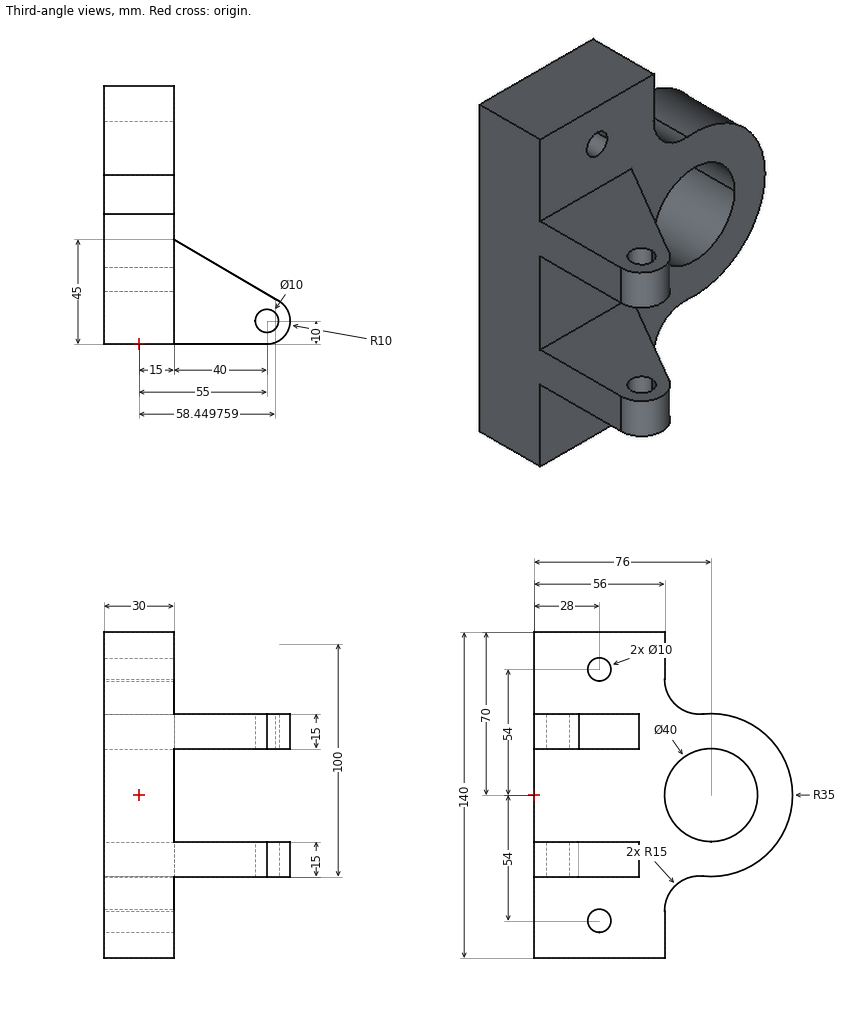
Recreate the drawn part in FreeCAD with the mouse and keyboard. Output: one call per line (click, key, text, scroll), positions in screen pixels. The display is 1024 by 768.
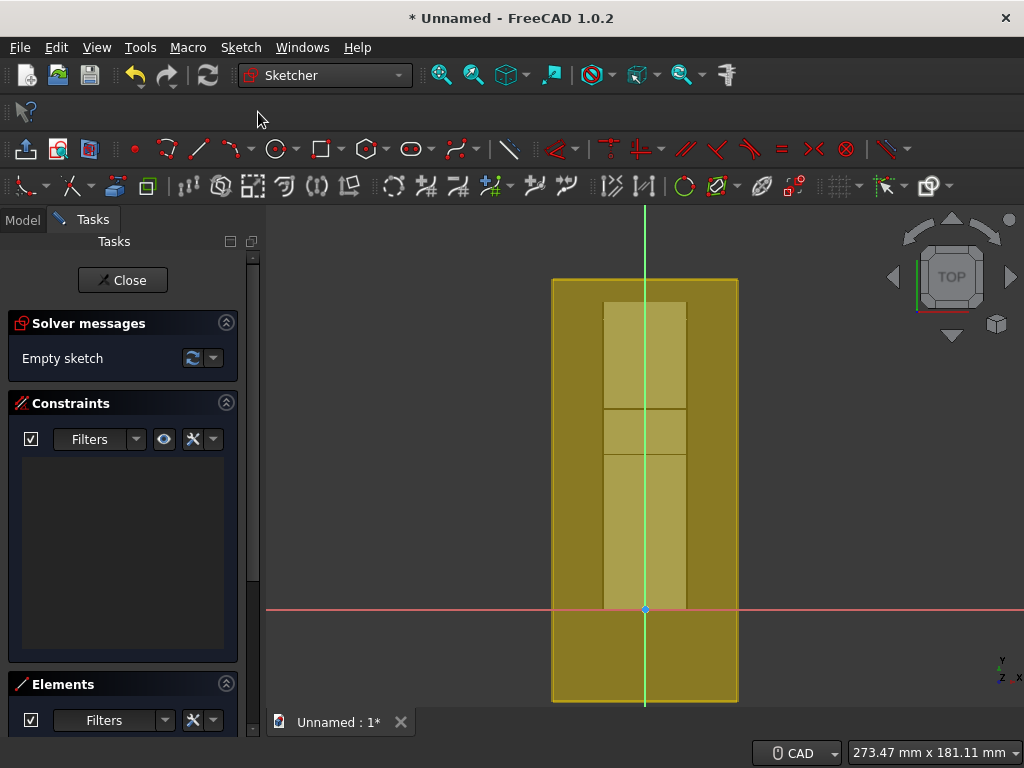
scroll(859, 622, up, 4)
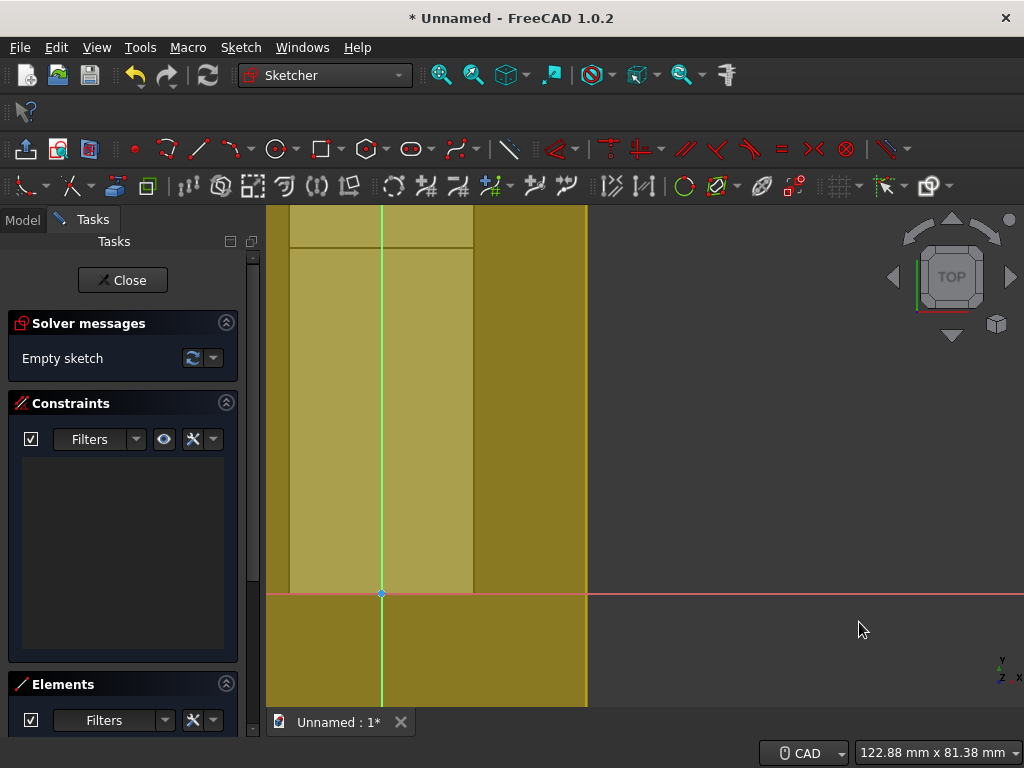
click(168, 150)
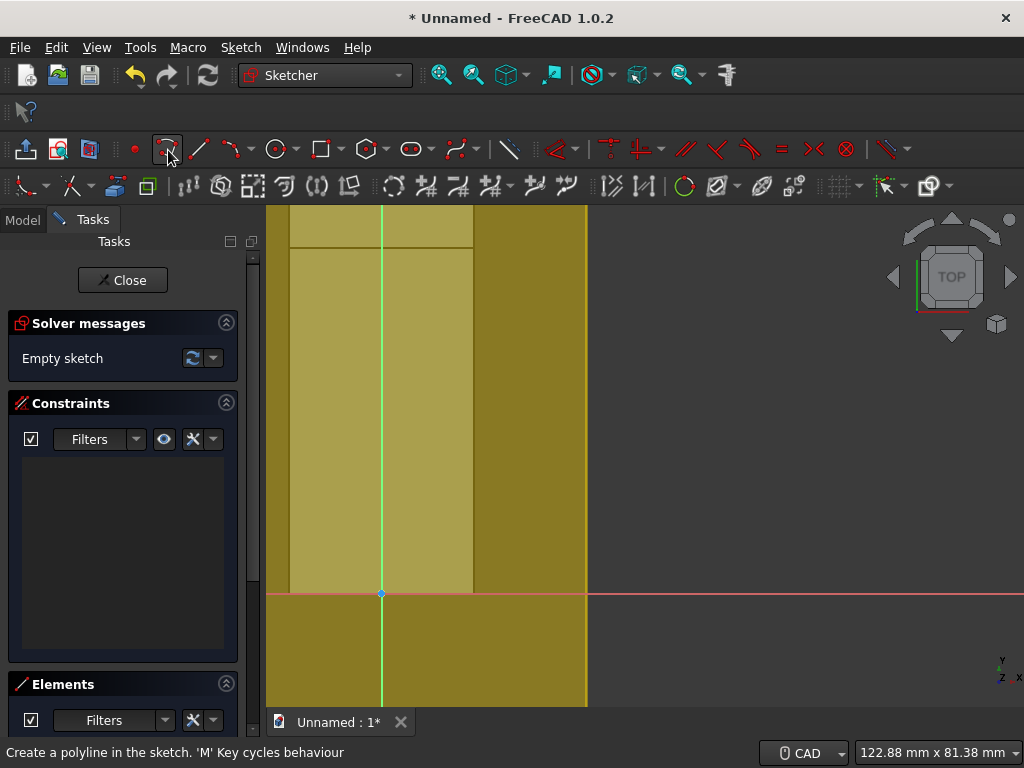
click(742, 474)
click(474, 316)
click(474, 594)
click(721, 585)
right_click(721, 585)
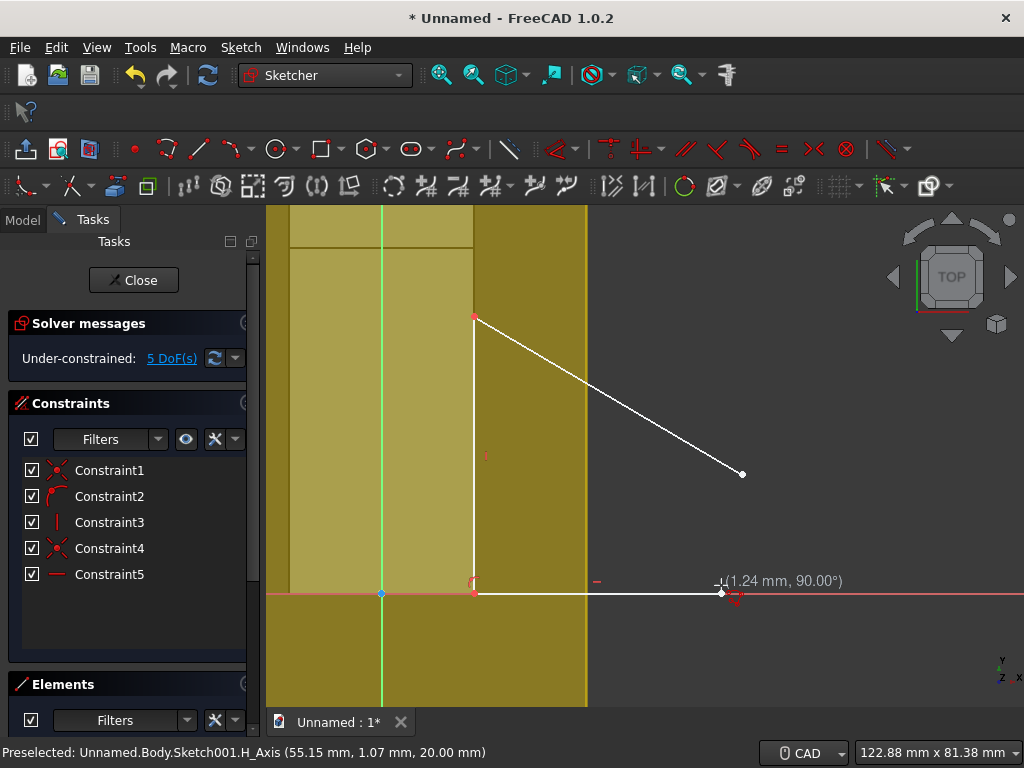
key(g)
key(3)
key(a)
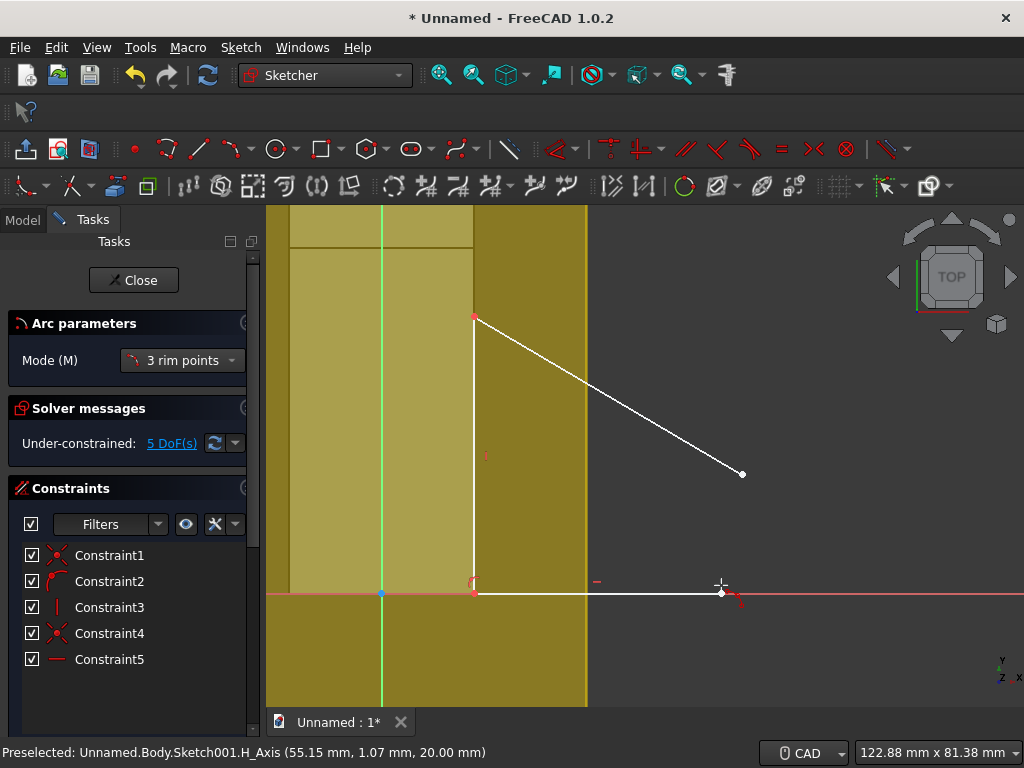
click(721, 594)
click(742, 475)
click(782, 543)
key(Escape)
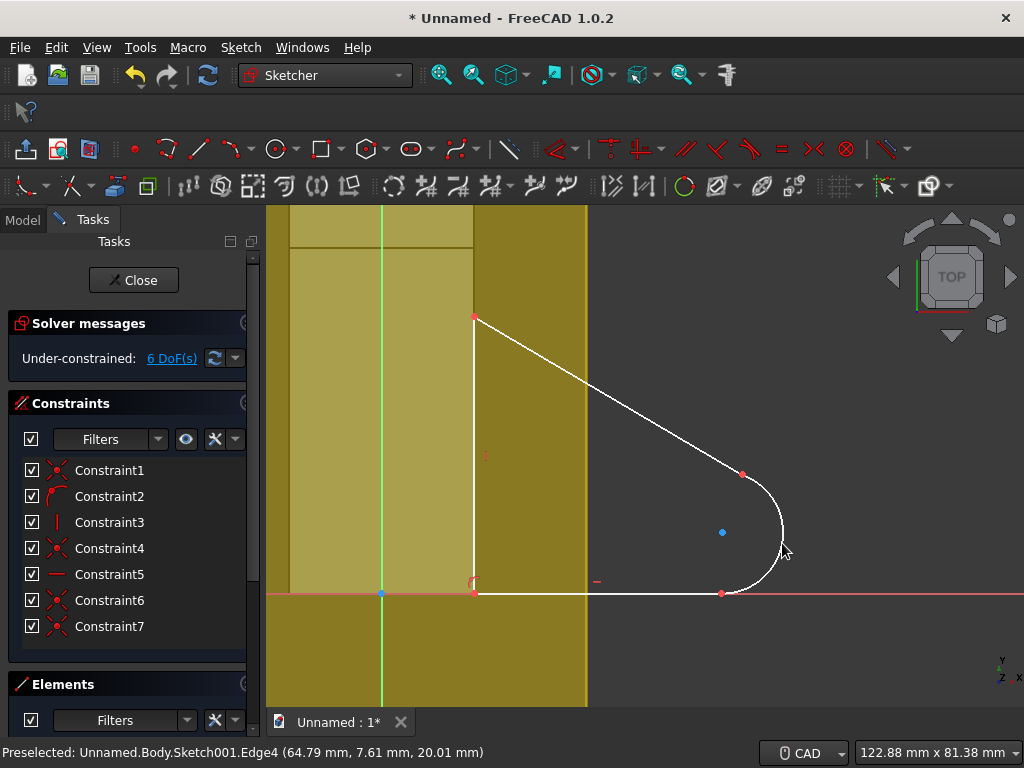
click(548, 594)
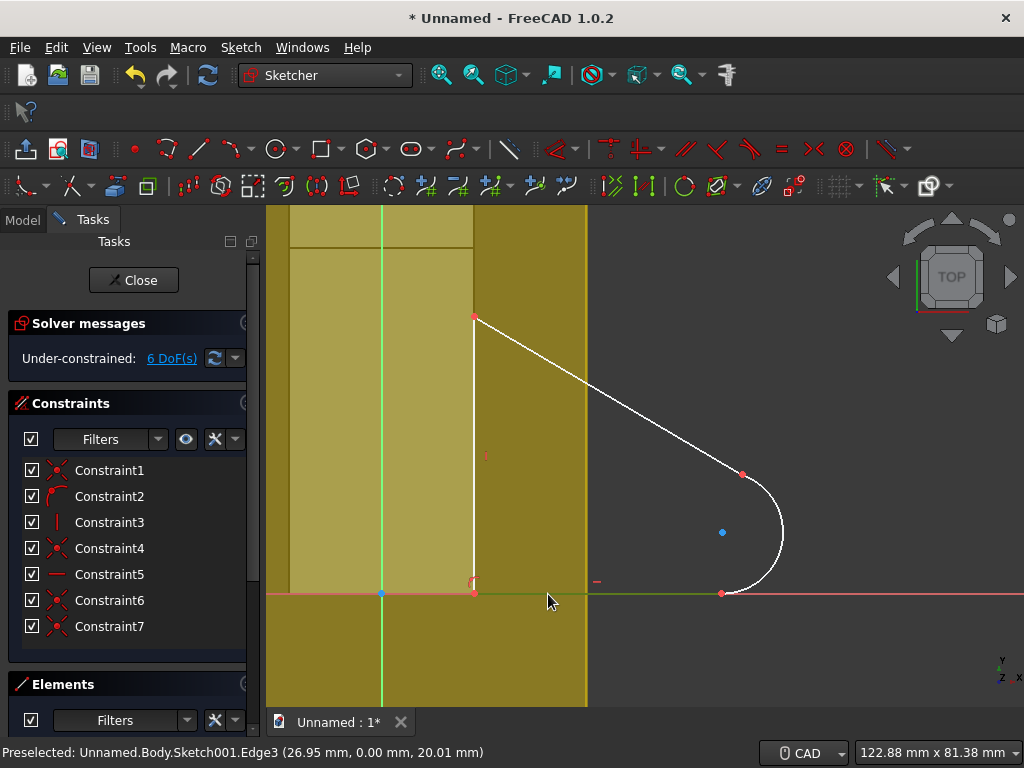
click(767, 574)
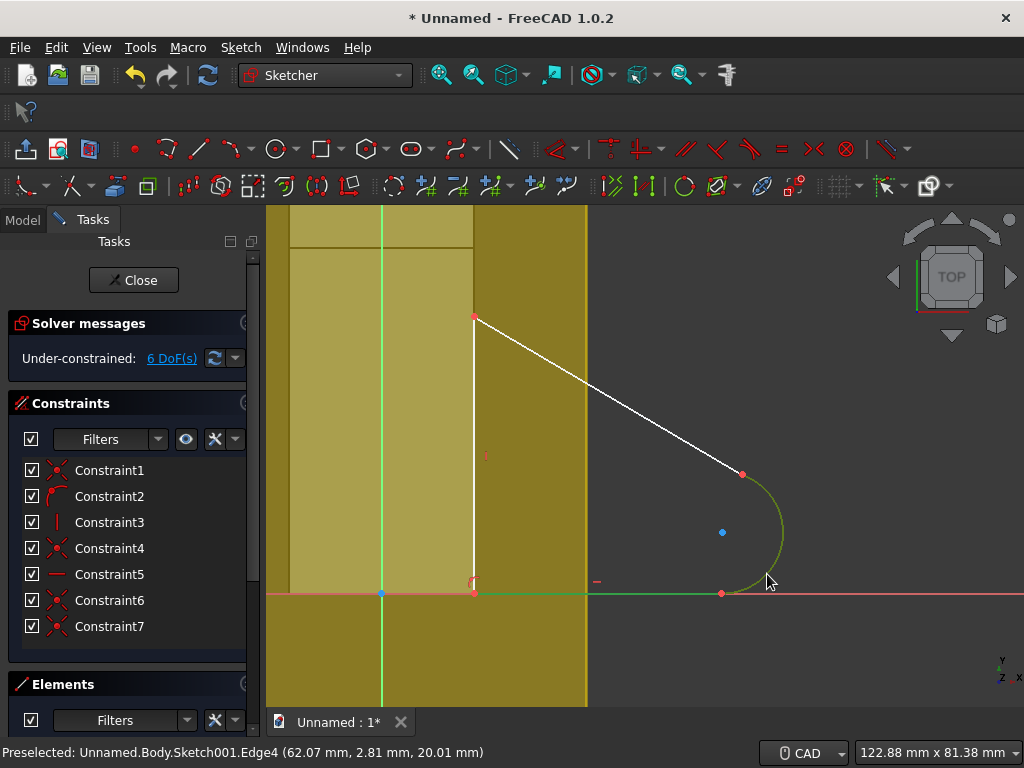
key(t)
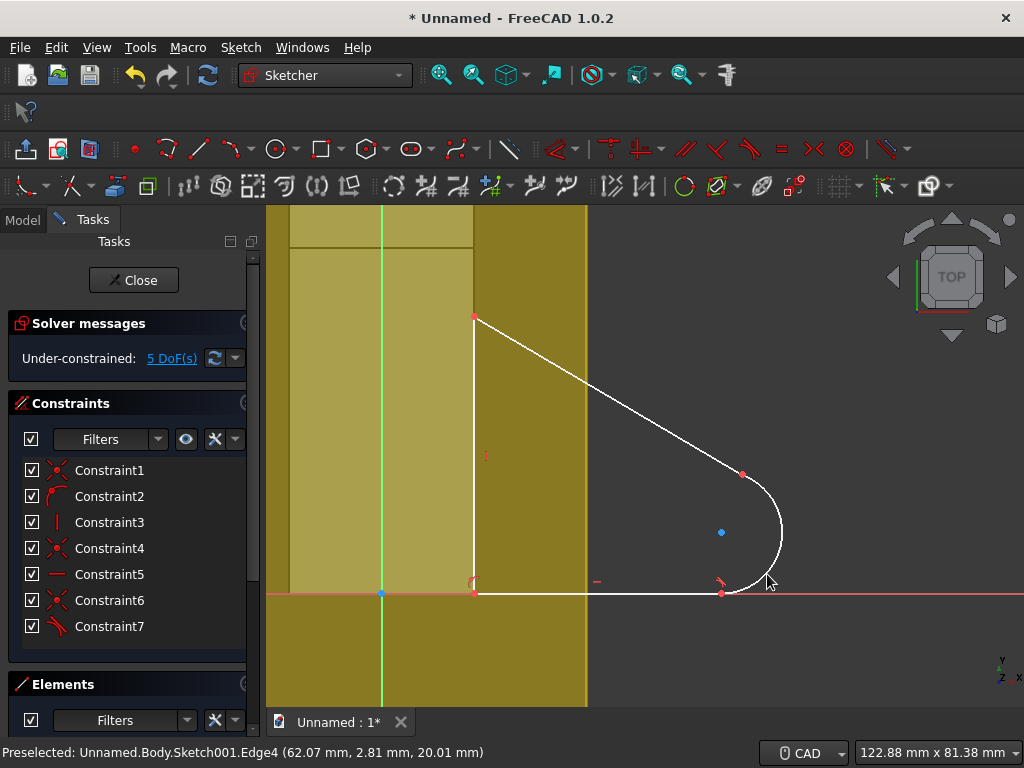
key(d)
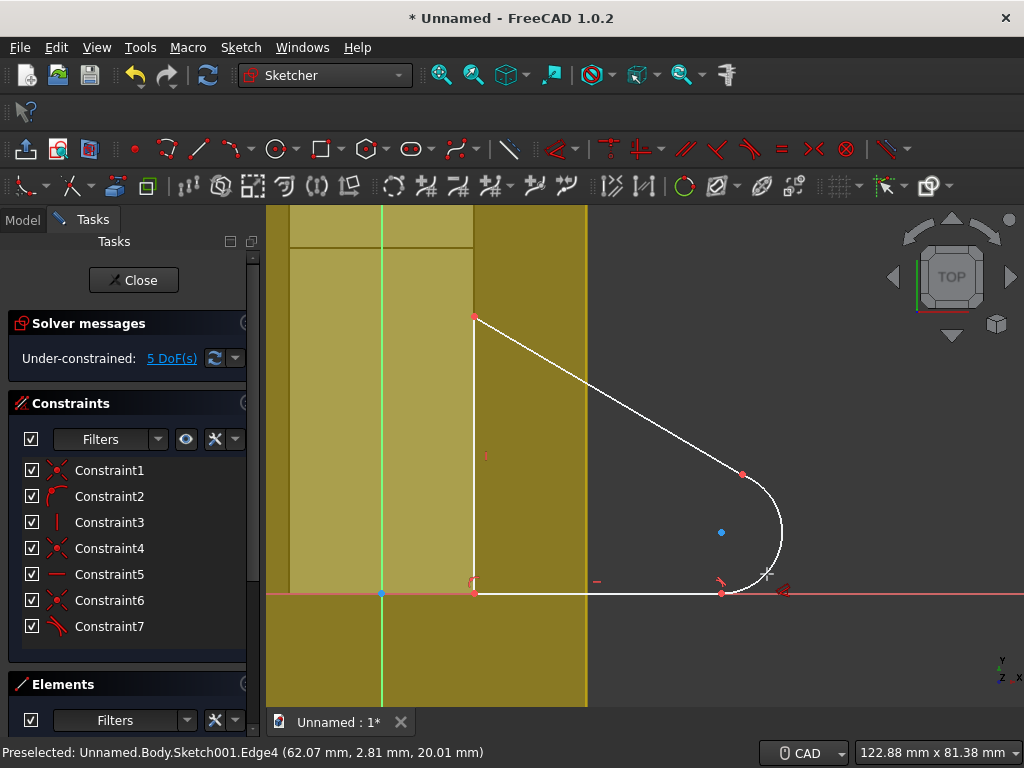
click(766, 573)
click(752, 620)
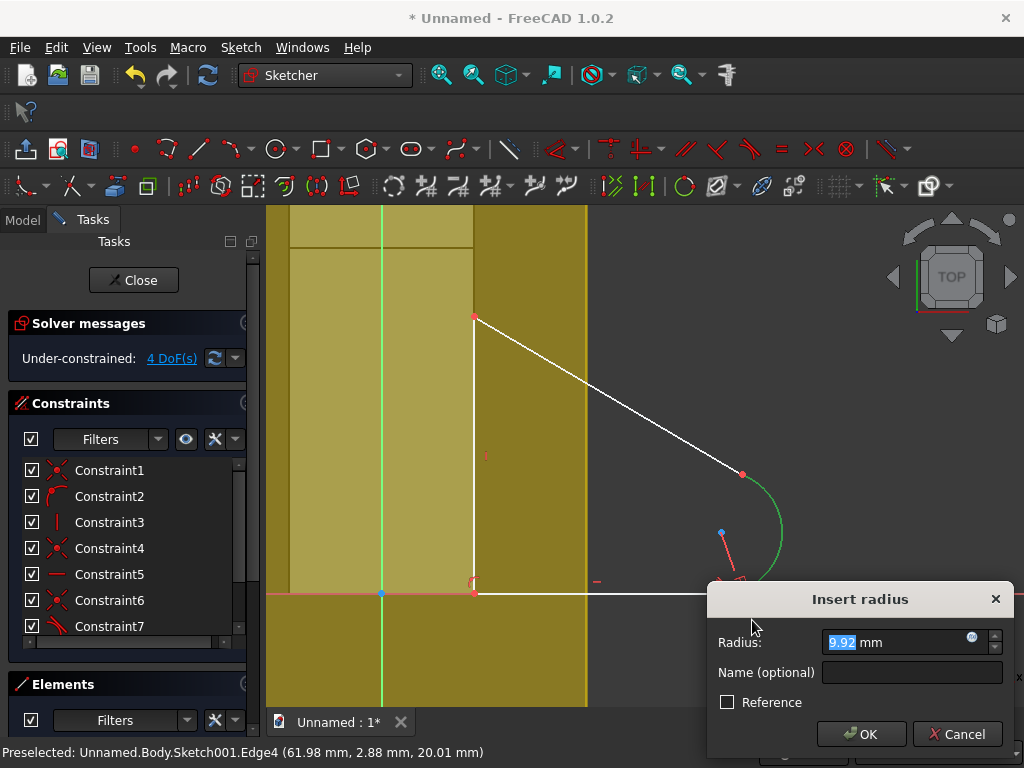
text(10)
key(Return)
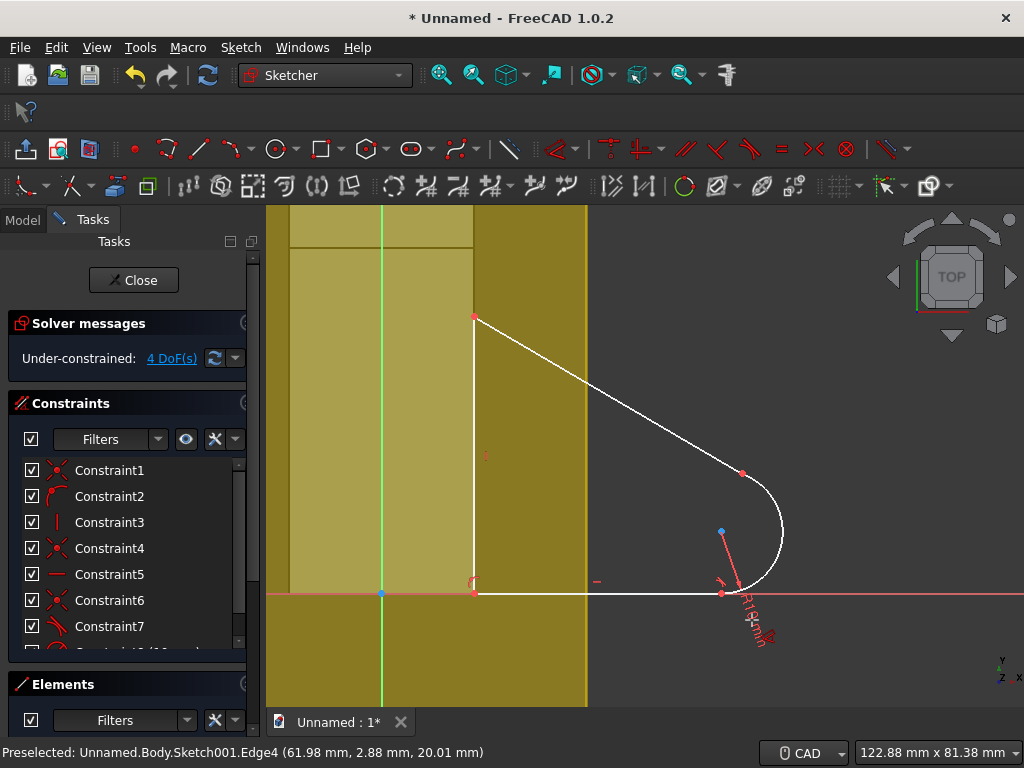
click(474, 400)
click(440, 455)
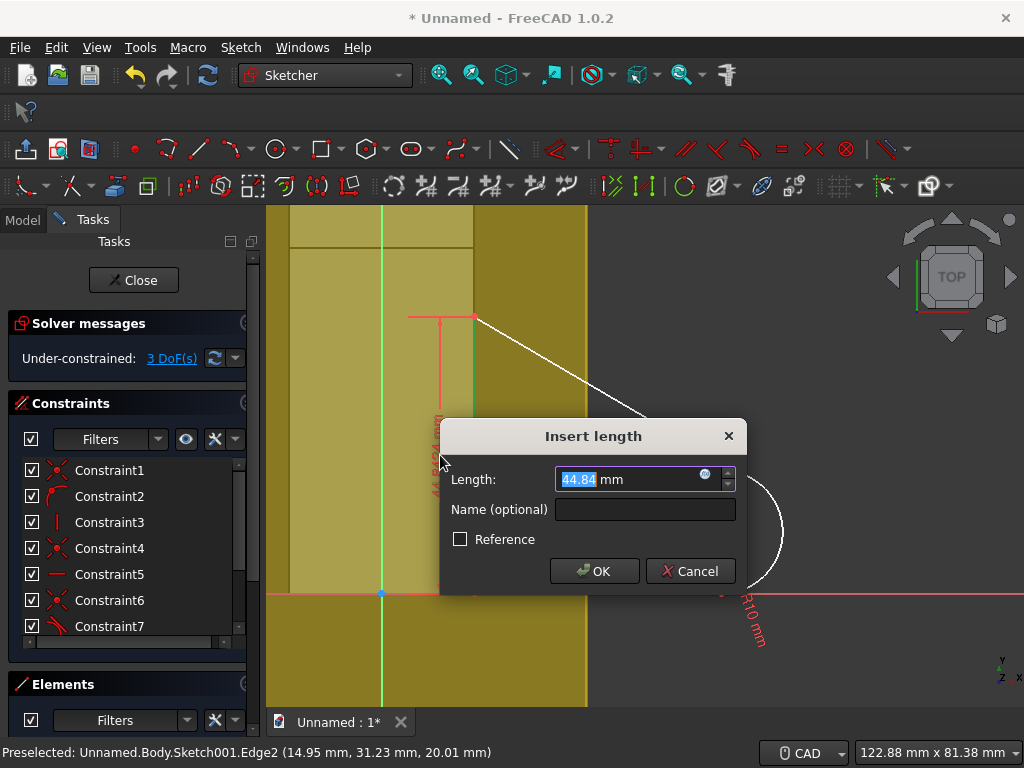
text(45)
key(Return)